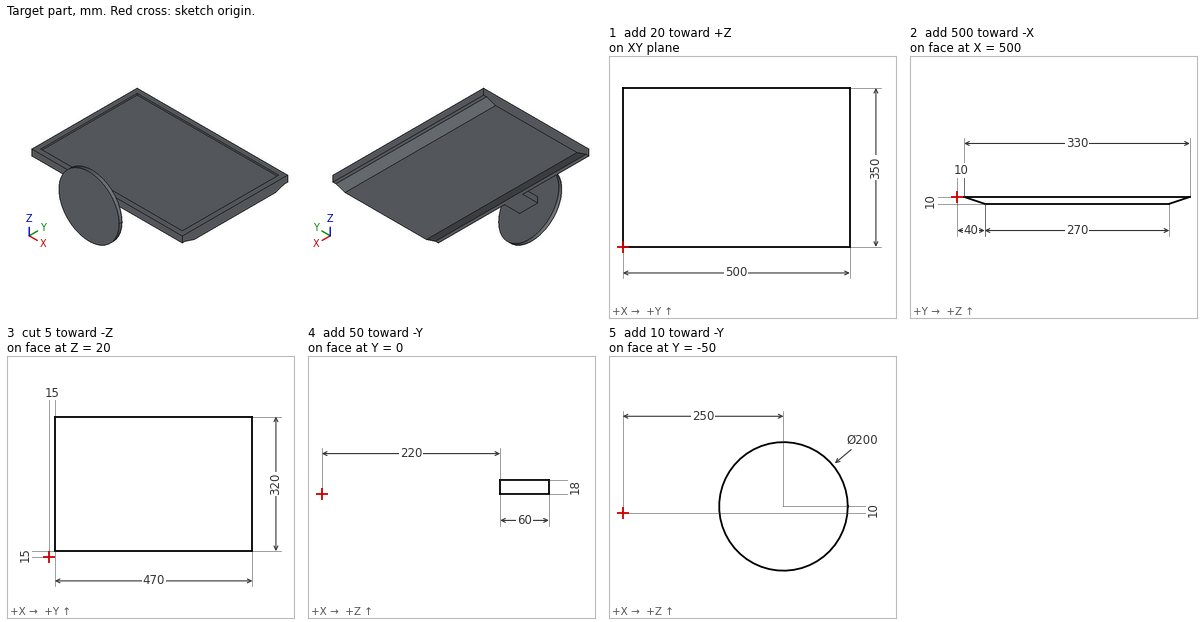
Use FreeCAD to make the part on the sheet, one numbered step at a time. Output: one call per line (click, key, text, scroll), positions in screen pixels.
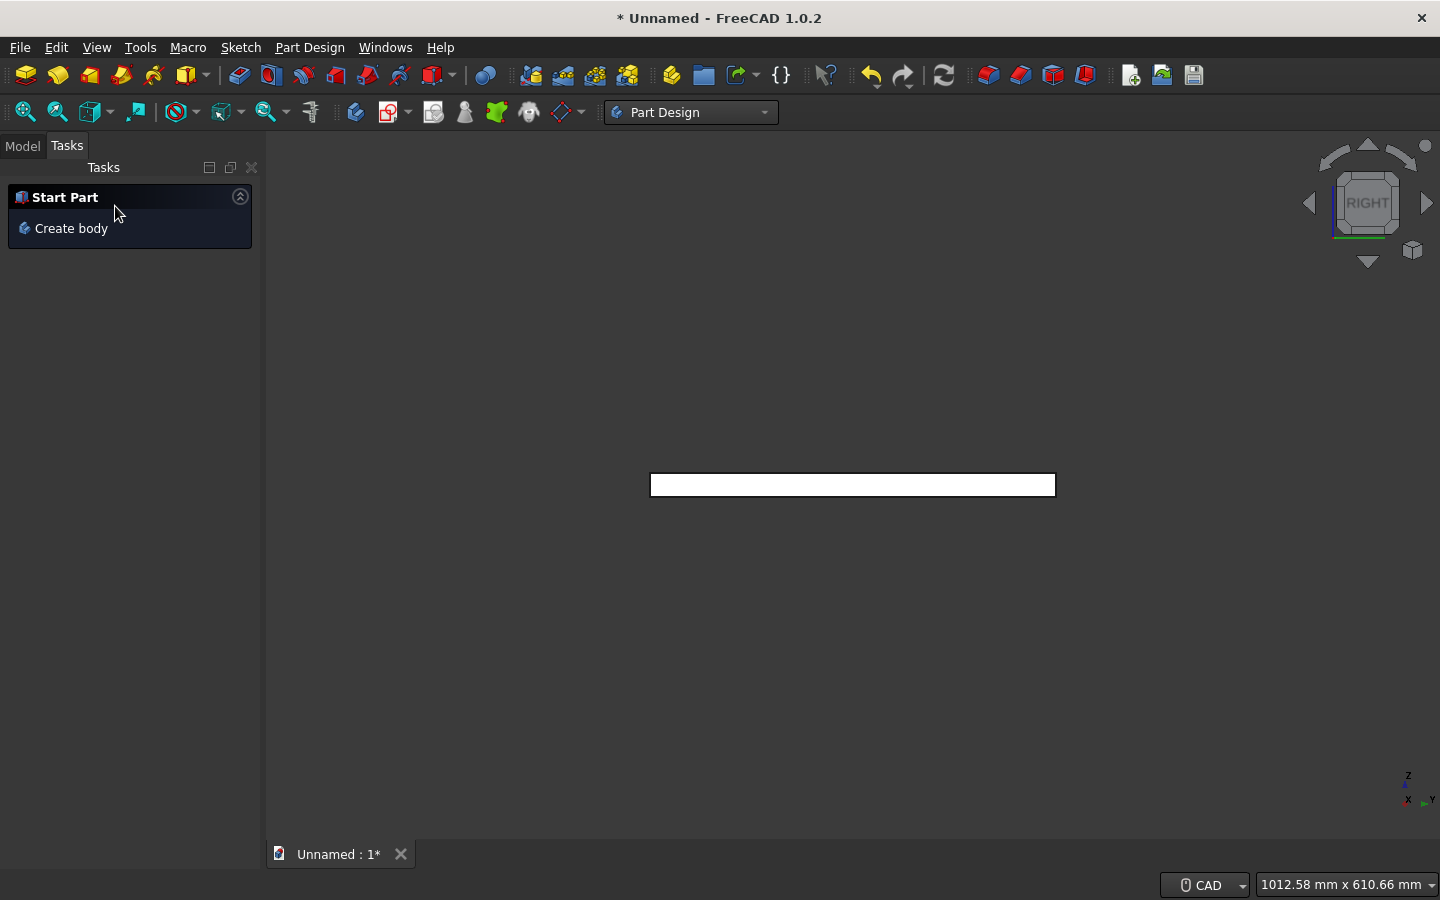
click(1027, 484)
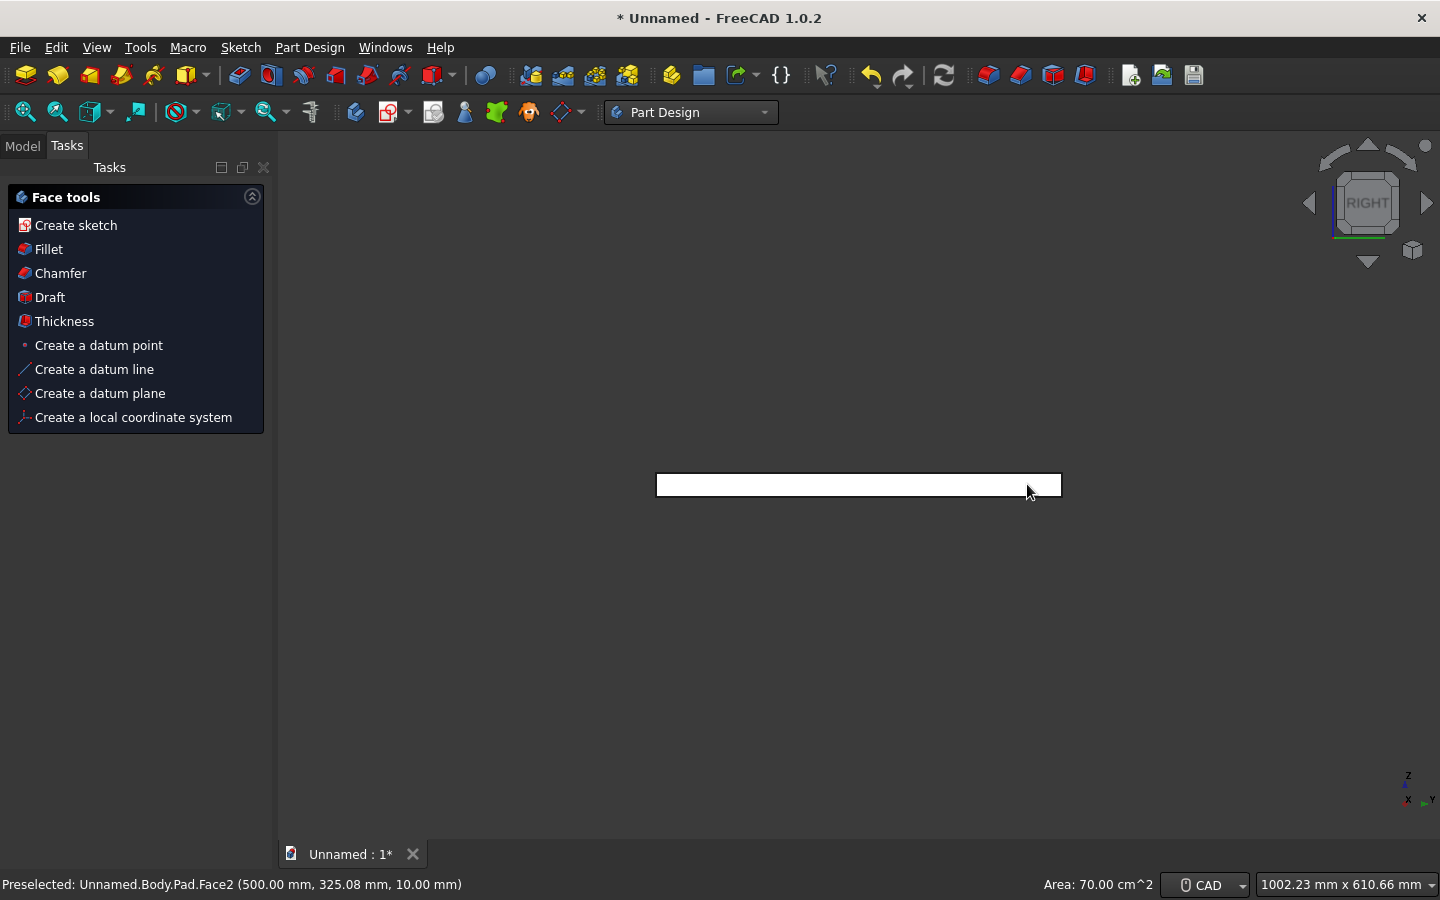
click(388, 112)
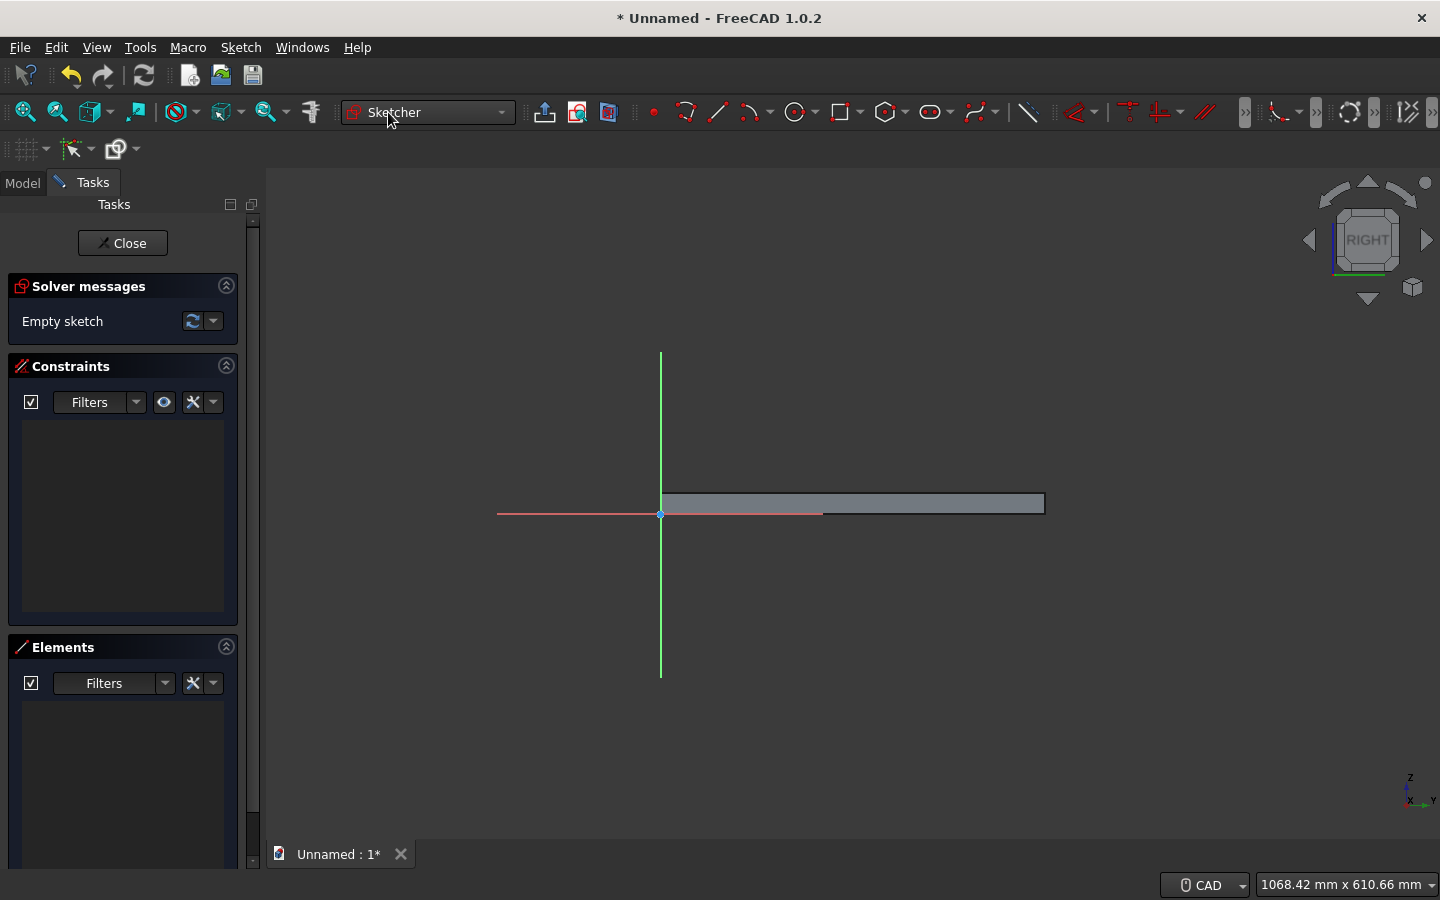
scroll(924, 540, up, 3)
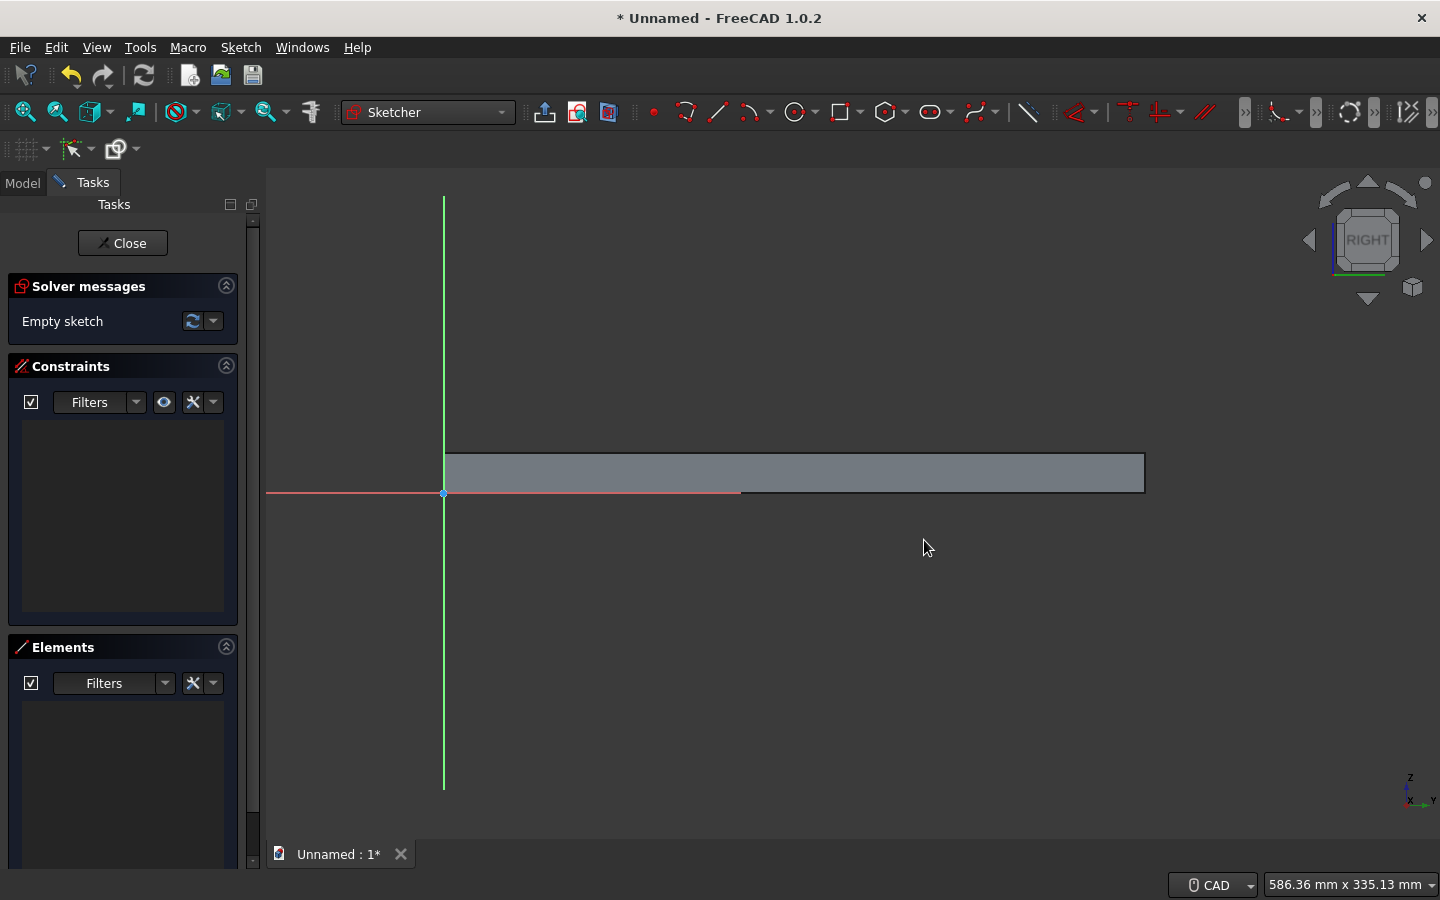
key(g)
key(m)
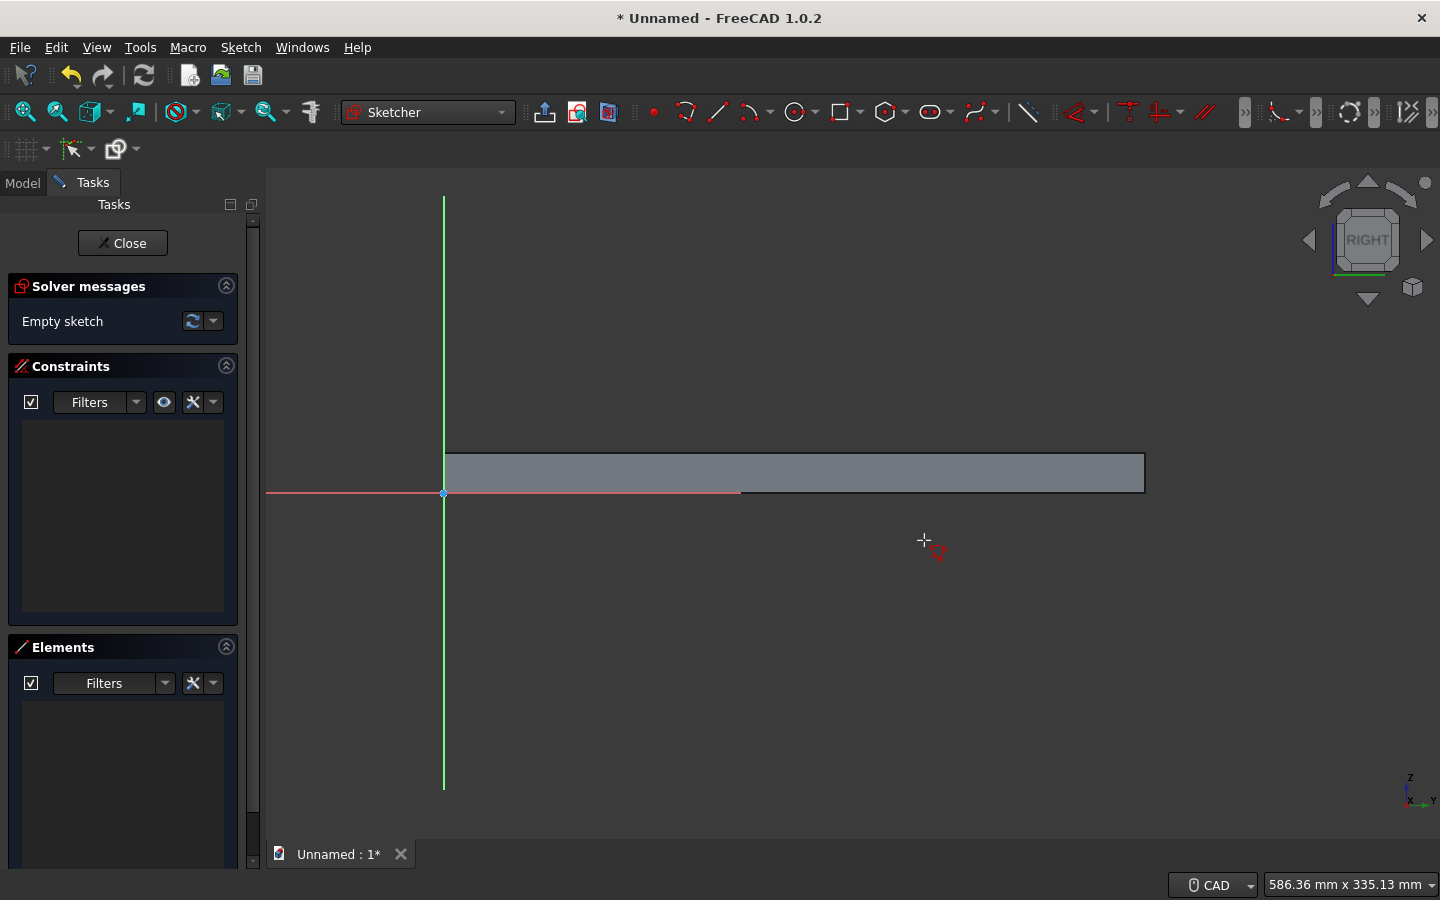
click(464, 493)
click(524, 513)
click(1064, 513)
click(1125, 502)
click(464, 493)
key(Escape)
key(Escape)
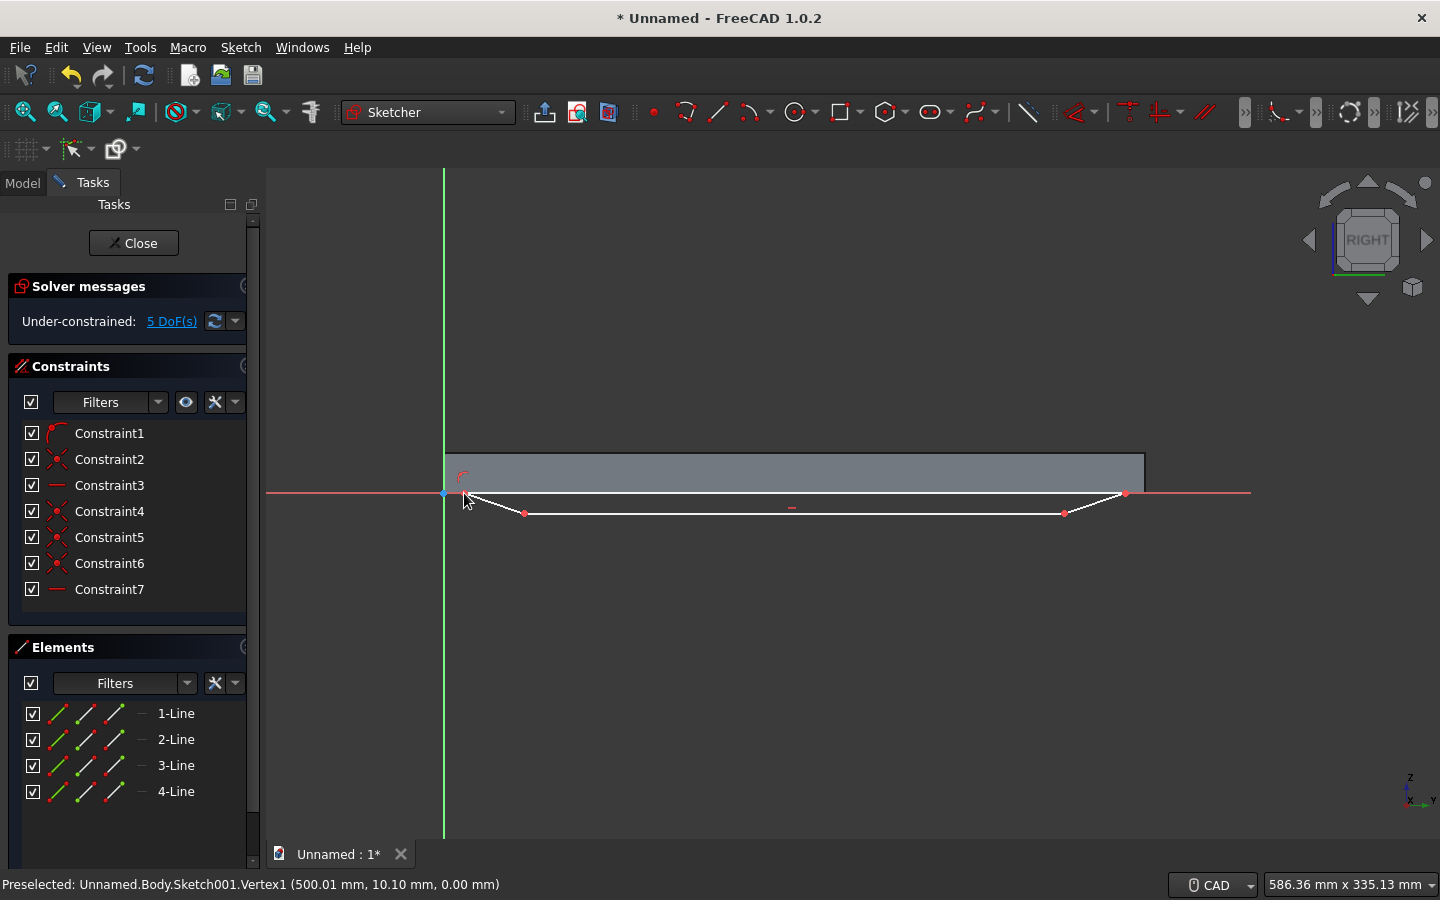
key(d)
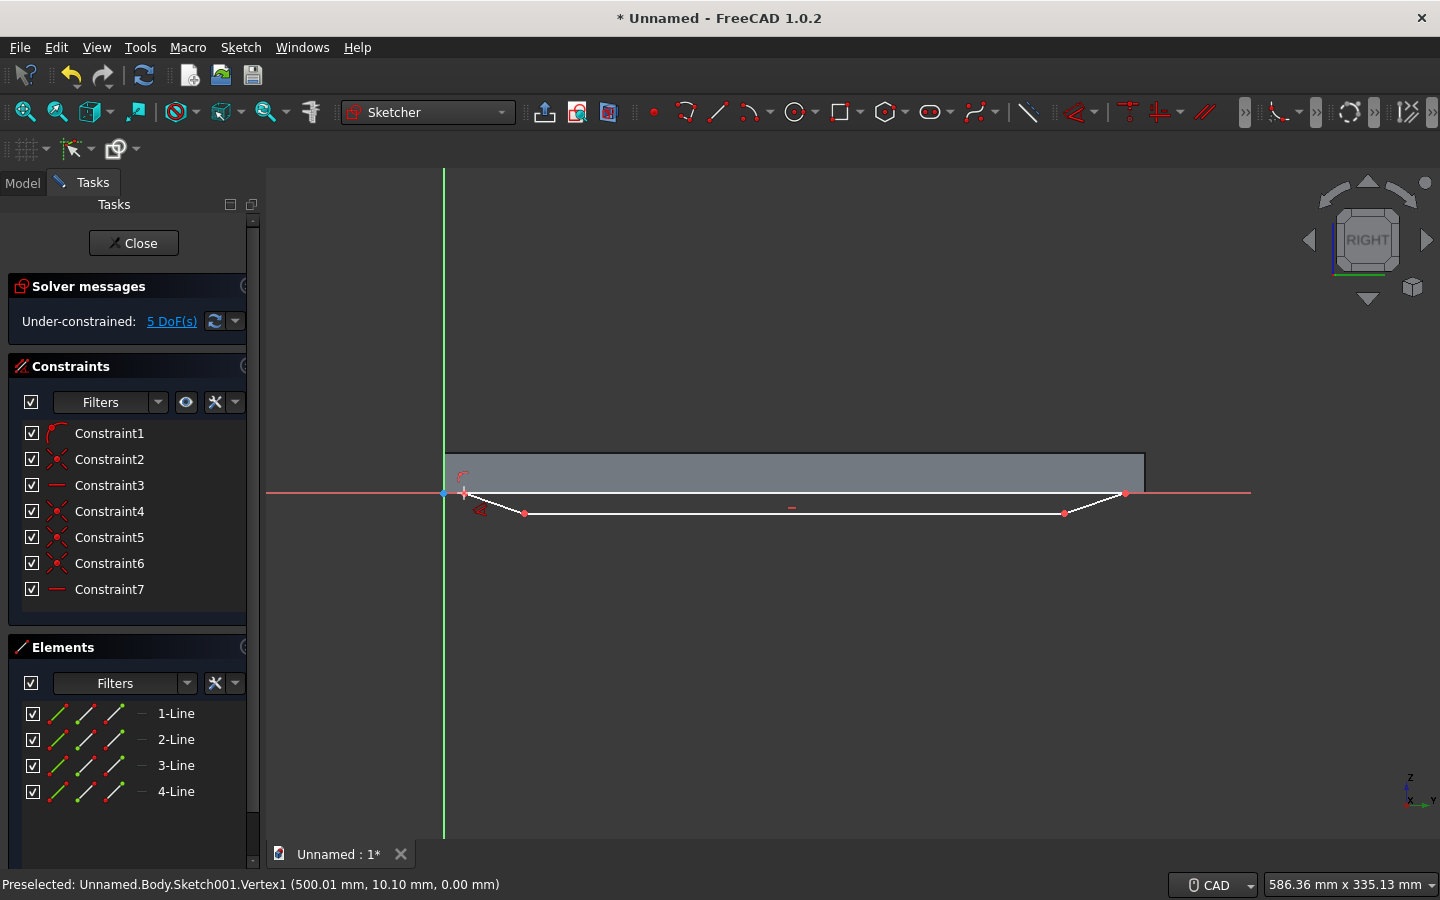
click(686, 514)
click(794, 548)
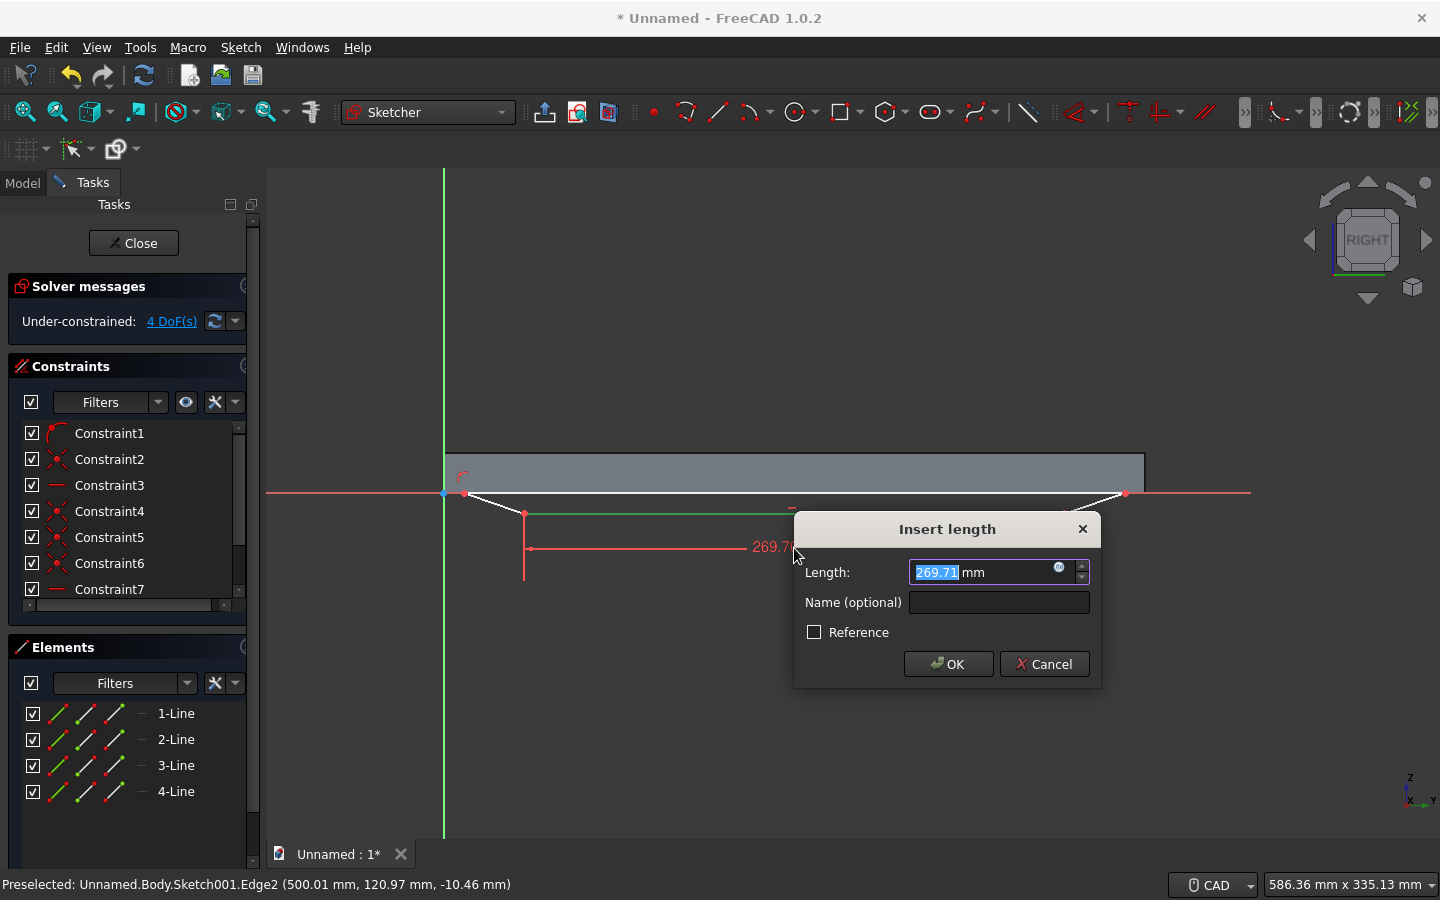
text(270)
key(Return)